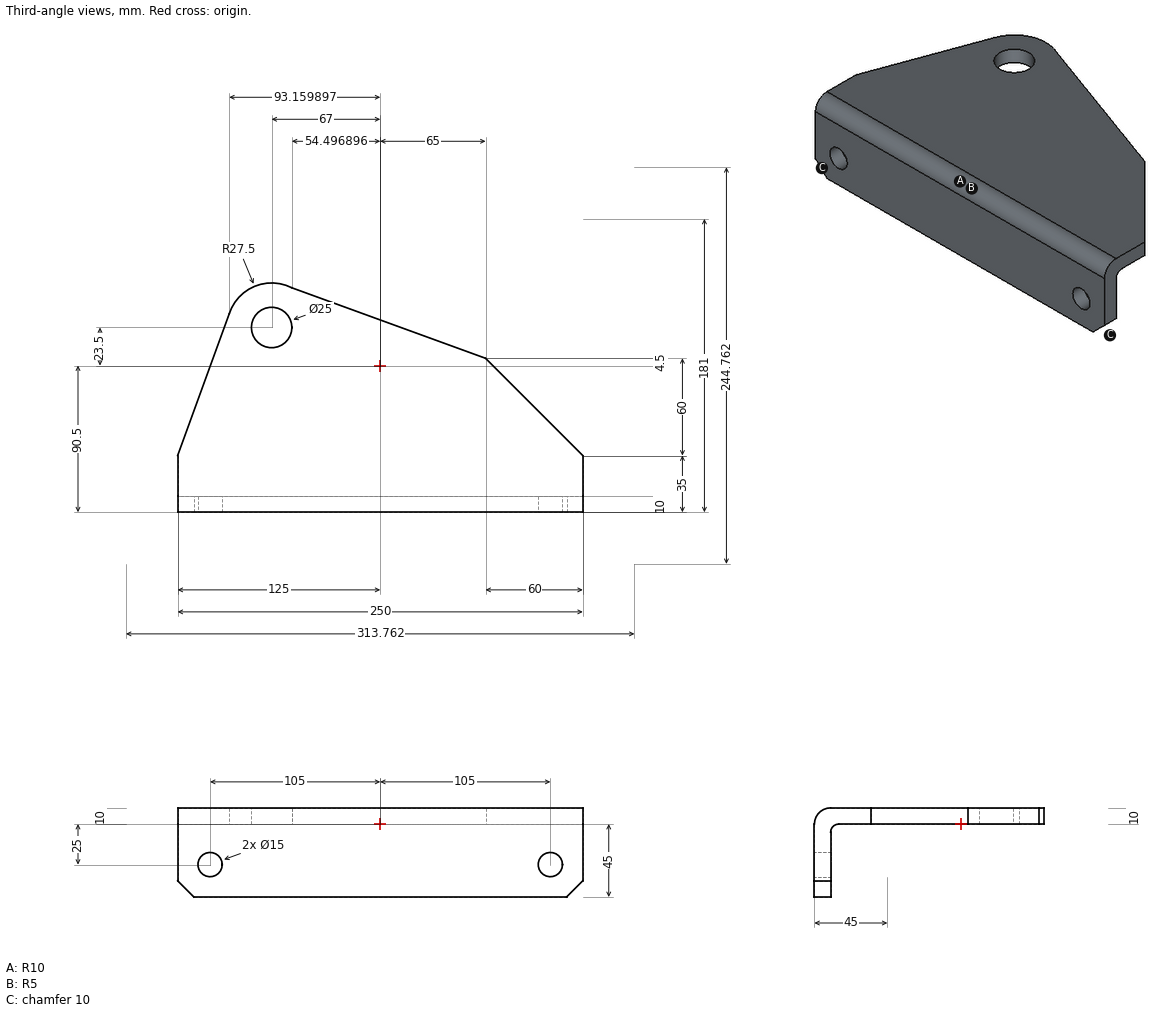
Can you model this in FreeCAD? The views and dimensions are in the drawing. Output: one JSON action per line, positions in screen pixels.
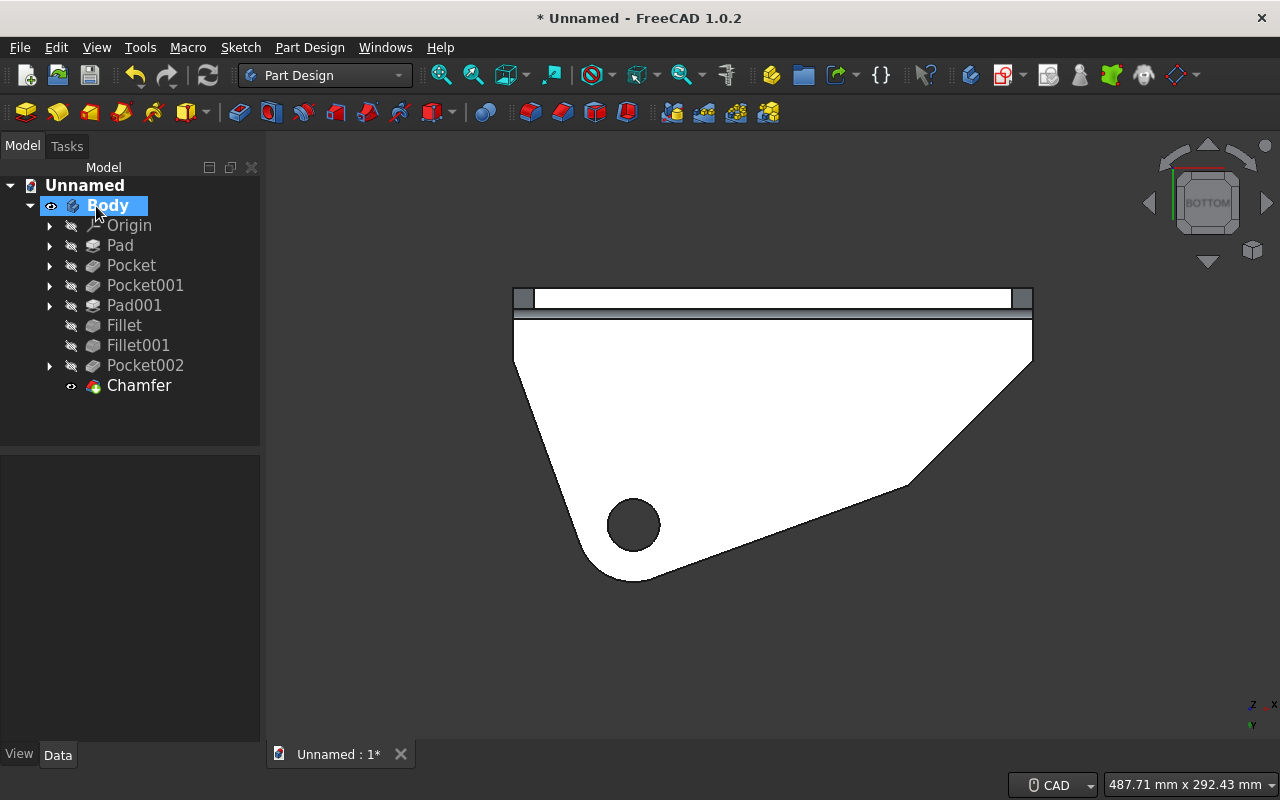
{"action": "key", "text": "0"}